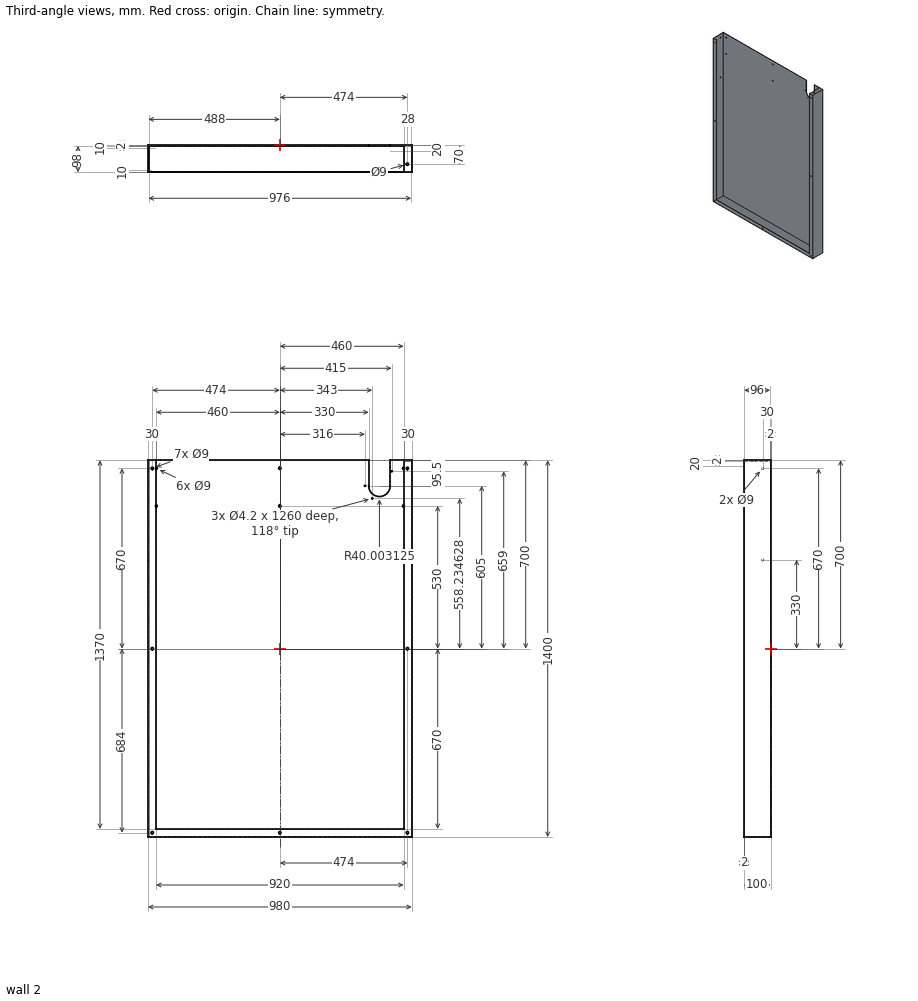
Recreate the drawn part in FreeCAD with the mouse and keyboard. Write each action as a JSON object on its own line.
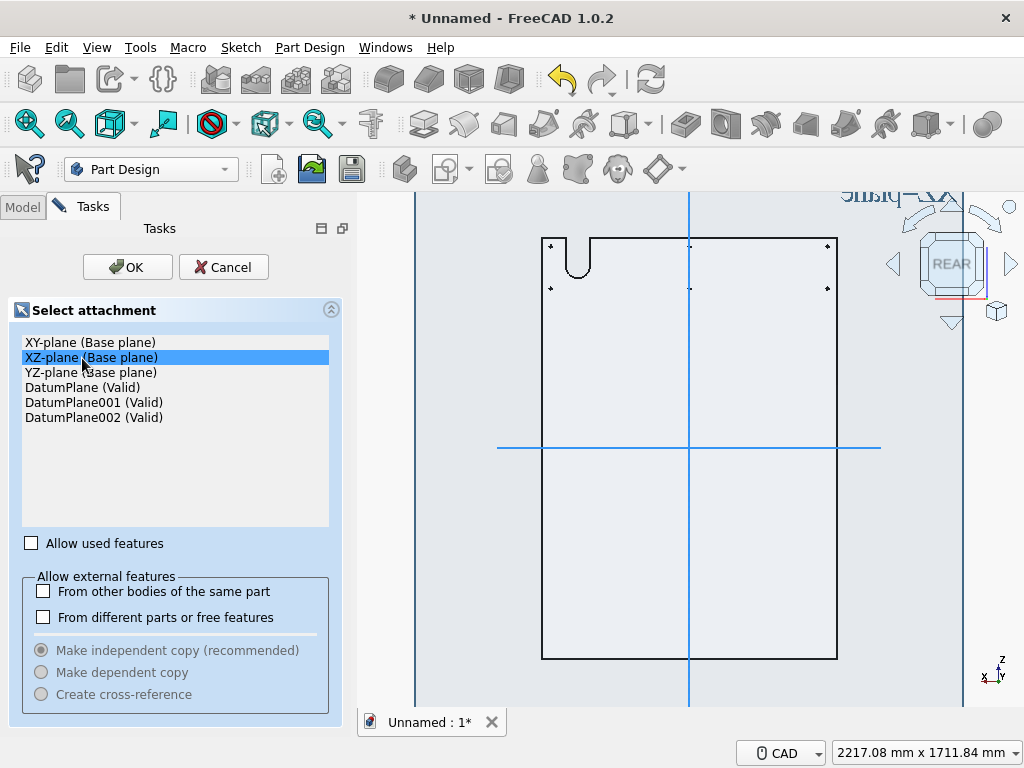
{"action": "left_click", "coordinate": [128, 267]}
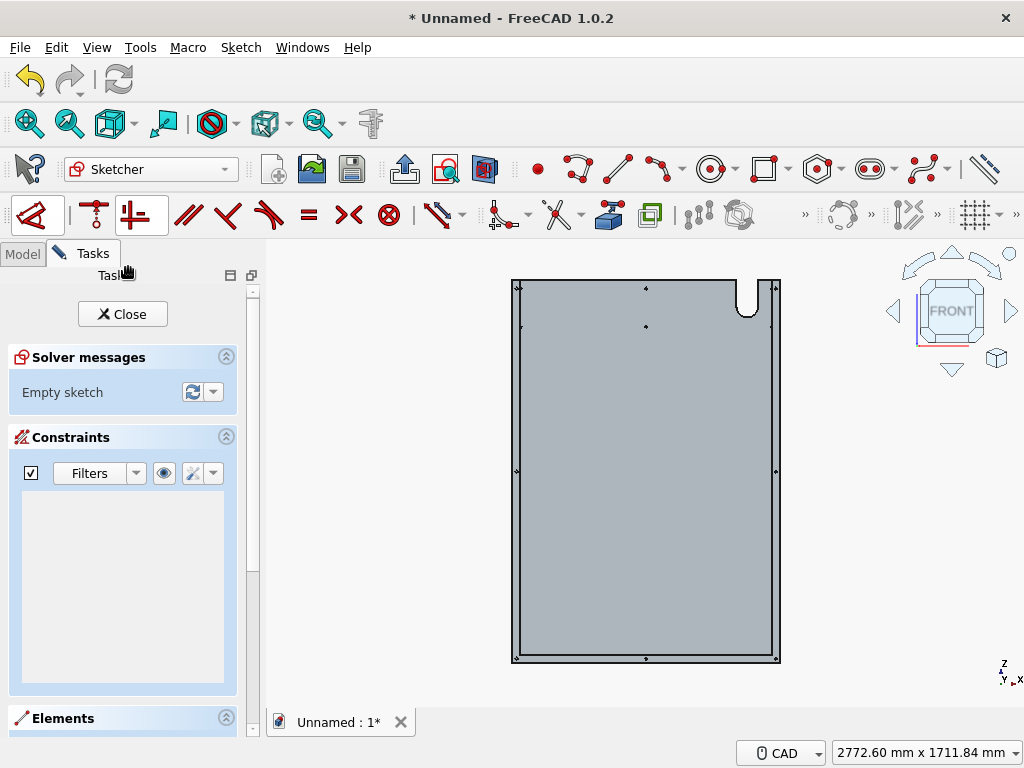
{"action": "left_click", "coordinate": [486, 170]}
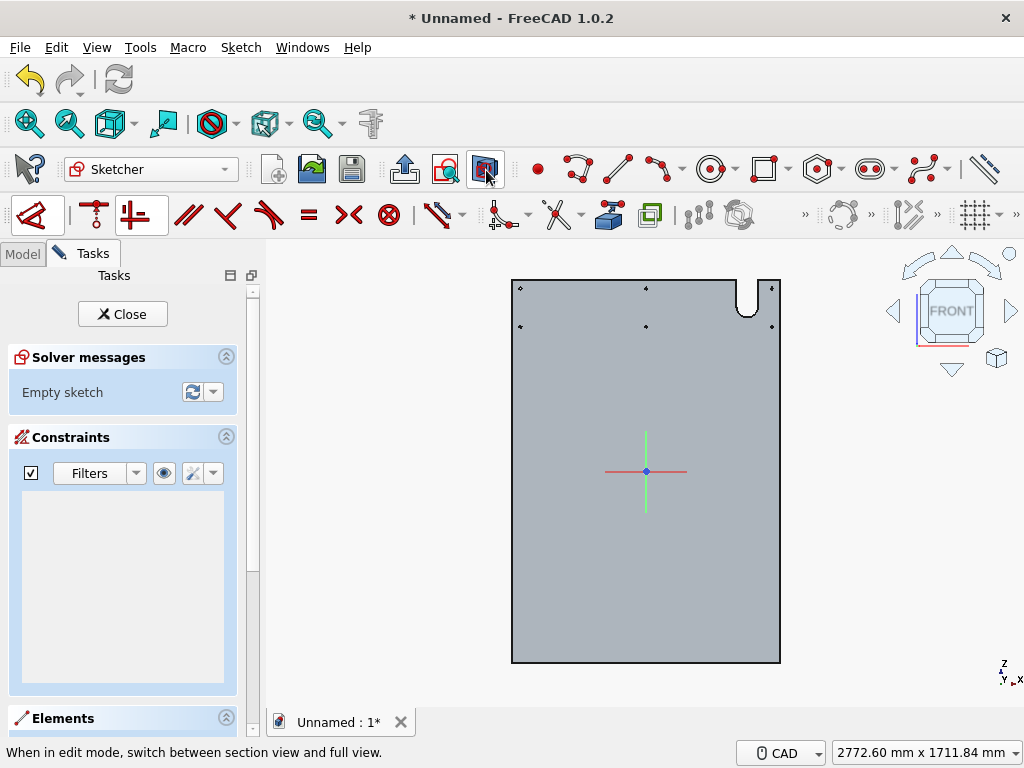
{"action": "scroll", "coordinate": [763, 289], "scroll_direction": "up", "scroll_amount": 12}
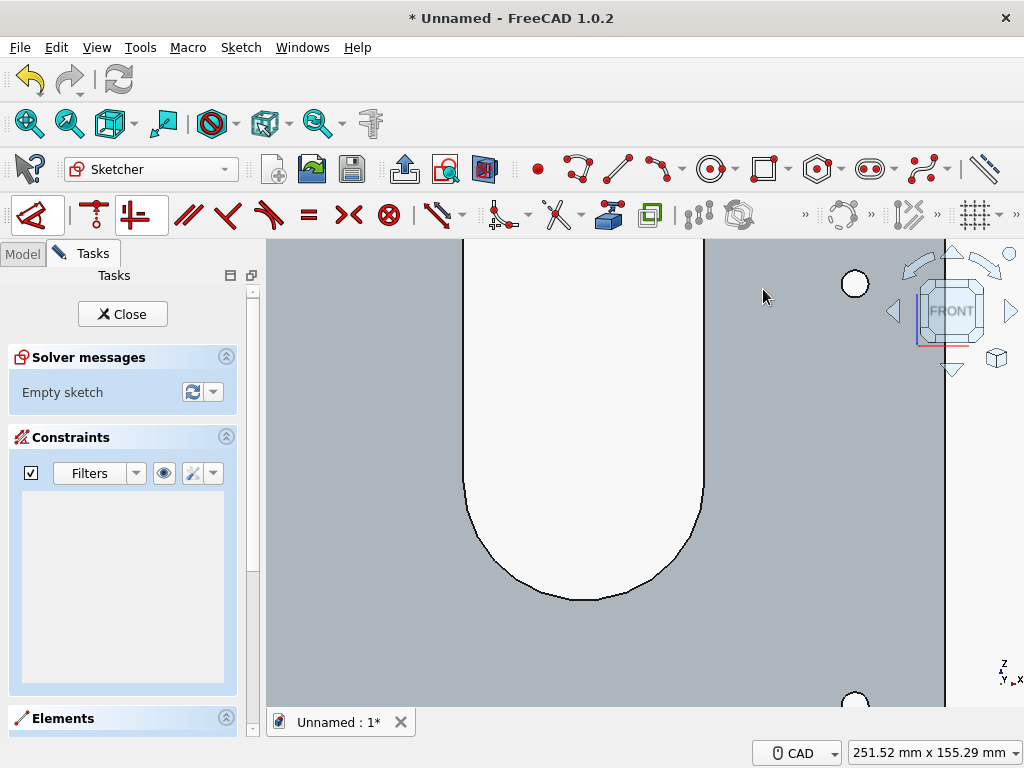
{"action": "left_click", "coordinate": [712, 170]}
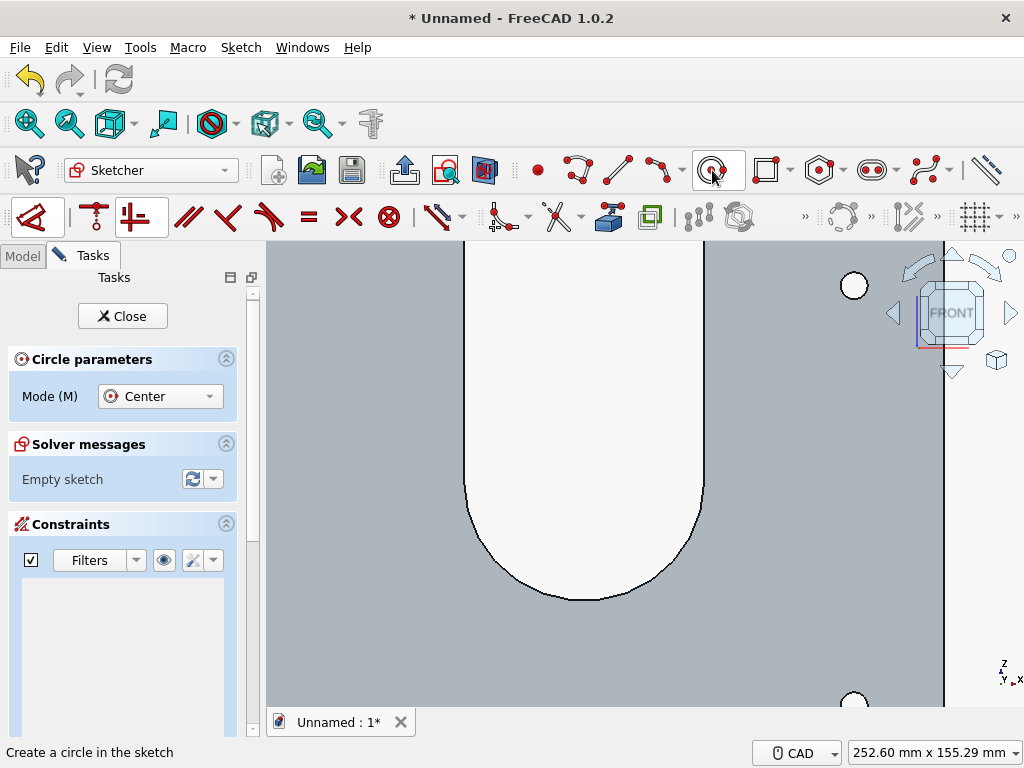
{"action": "scroll", "coordinate": [503, 621], "scroll_direction": "up", "scroll_amount": 7}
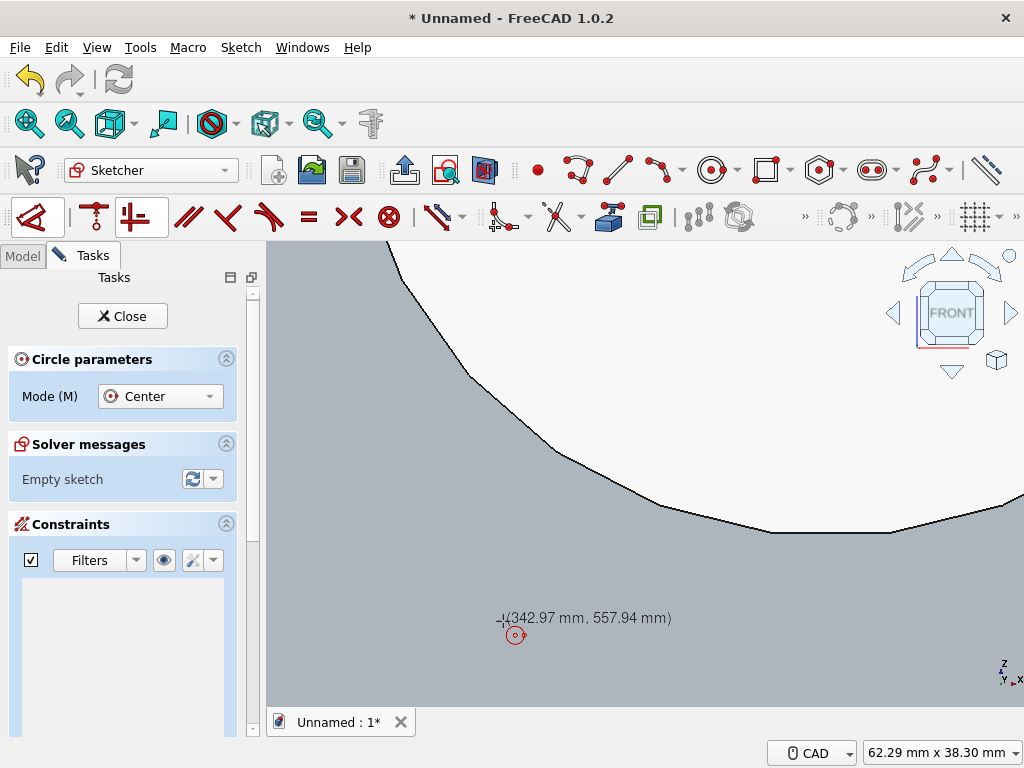
{"action": "scroll", "coordinate": [511, 627], "scroll_direction": "down", "scroll_amount": 7}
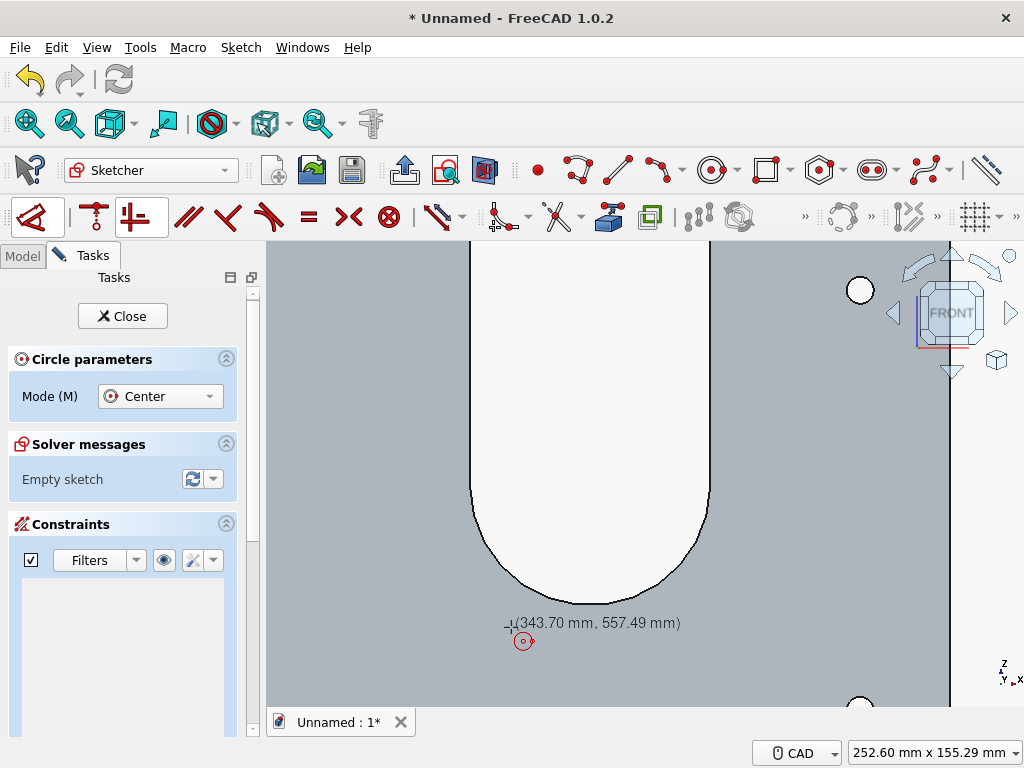
{"action": "left_click", "coordinate": [509, 626]}
{"action": "mouse_move", "coordinate": [514, 621]}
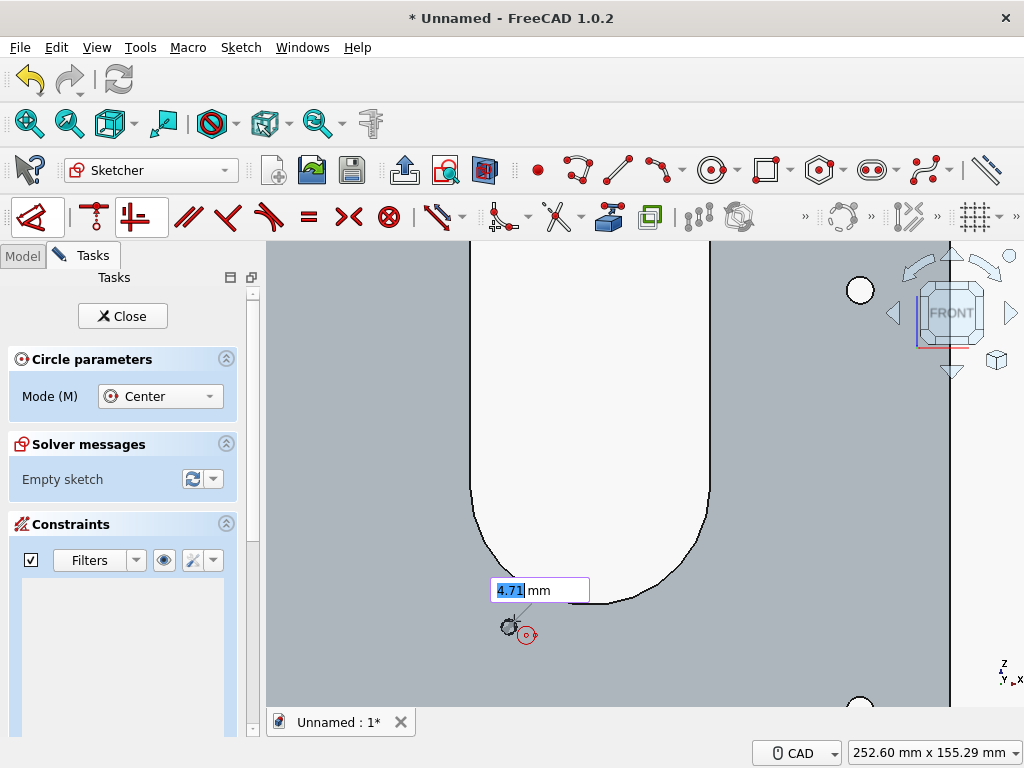
{"action": "type", "text": "4.2"}
{"action": "key", "text": "Return"}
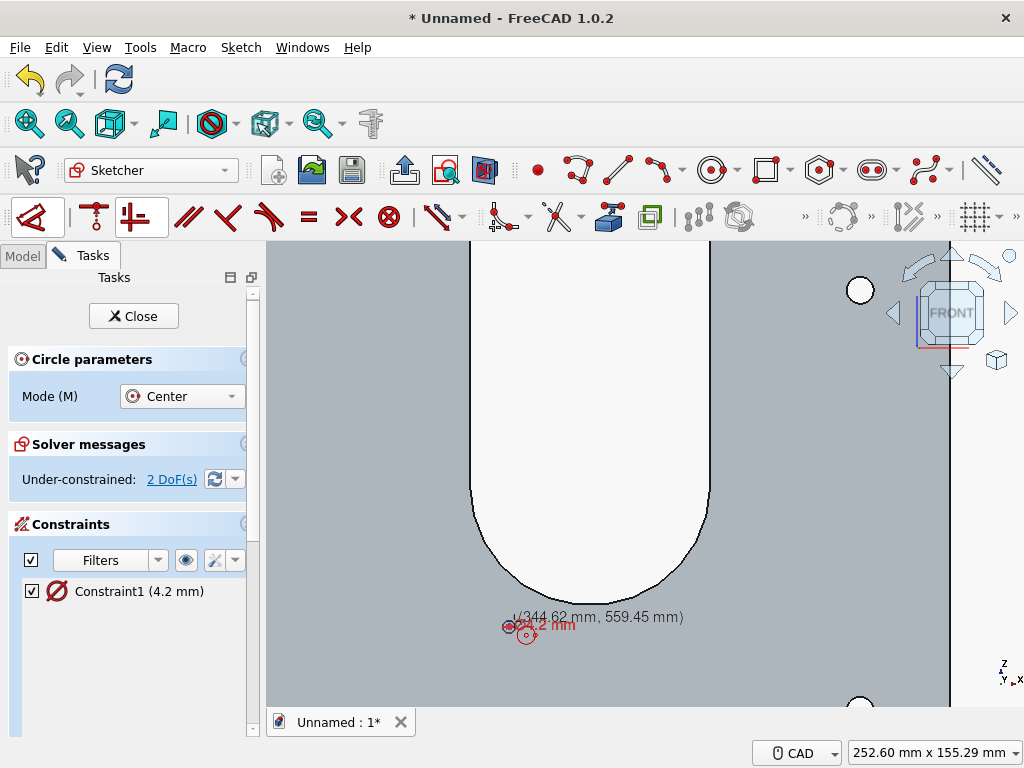
{"action": "scroll", "coordinate": [428, 485], "scroll_direction": "up", "scroll_amount": 7}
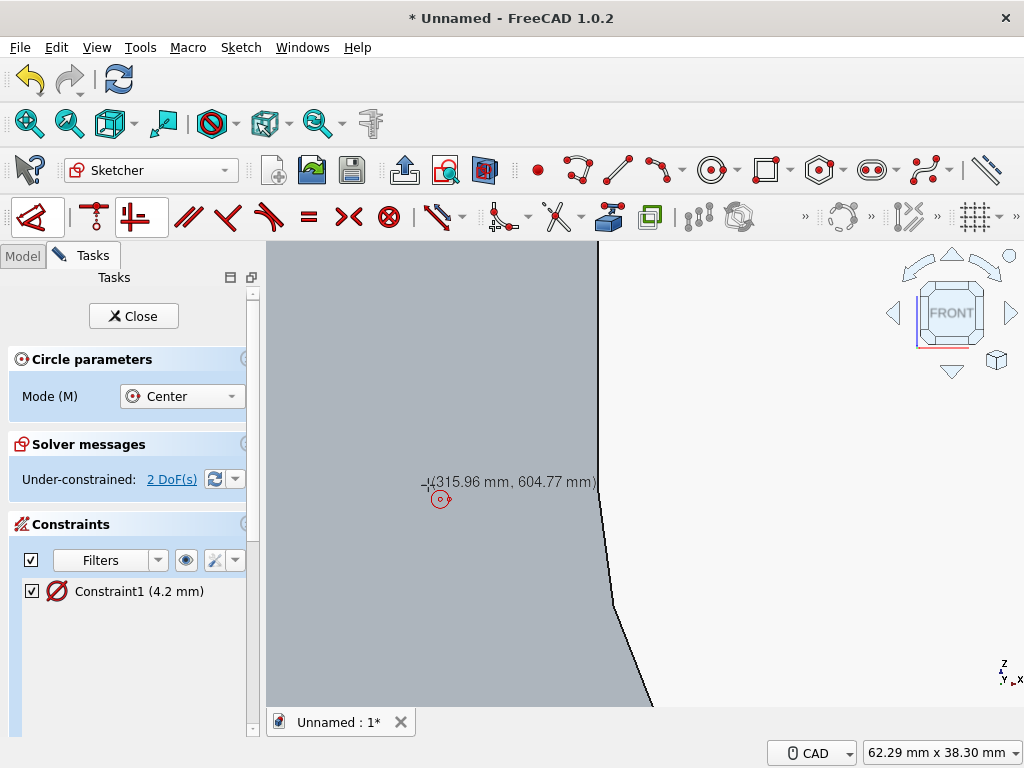
{"action": "scroll", "coordinate": [428, 485], "scroll_direction": "down", "scroll_amount": 7}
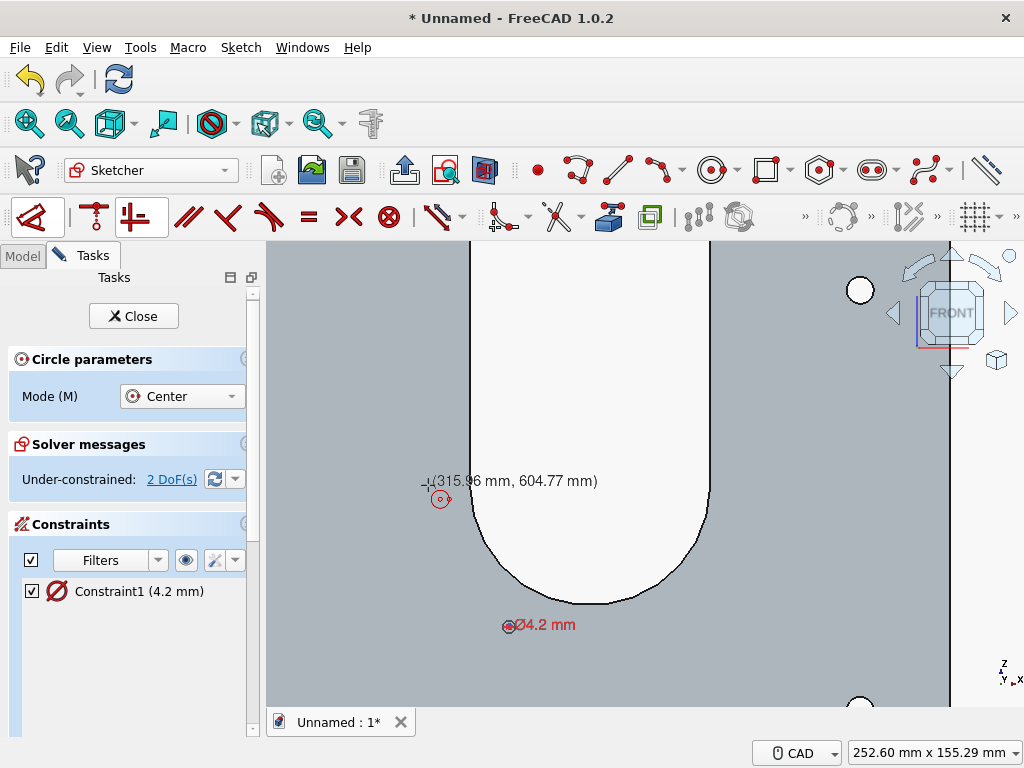
{"action": "left_click", "coordinate": [428, 485]}
{"action": "mouse_move", "coordinate": [433, 481]}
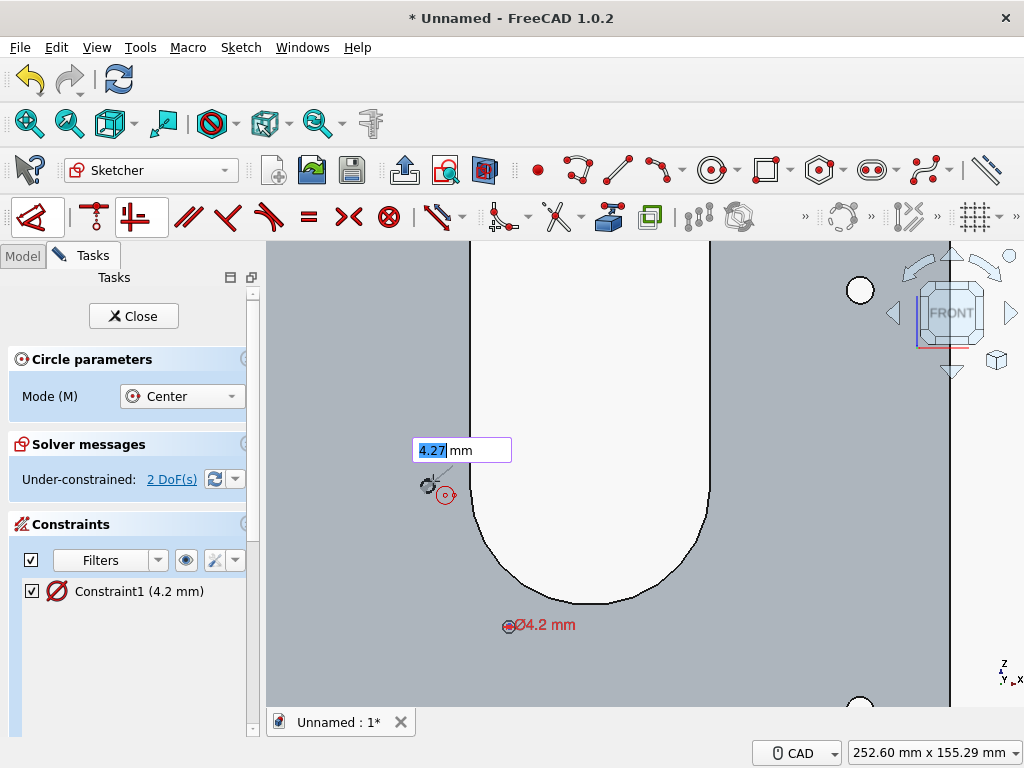
{"action": "type", "text": "4.2"}
{"action": "key", "text": "Return"}